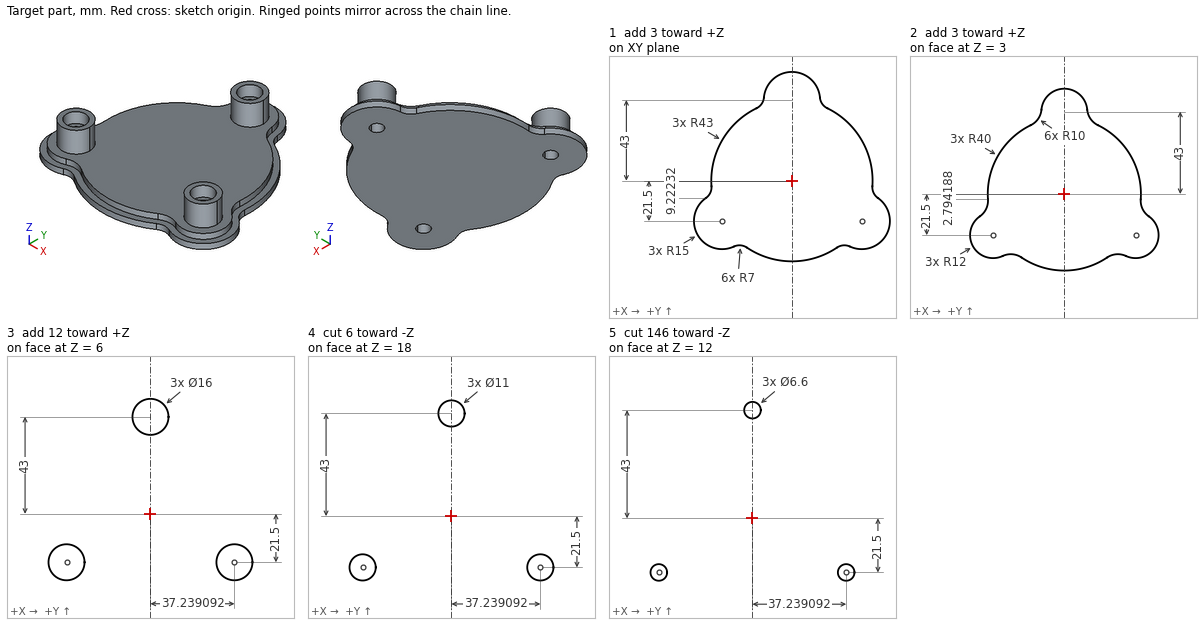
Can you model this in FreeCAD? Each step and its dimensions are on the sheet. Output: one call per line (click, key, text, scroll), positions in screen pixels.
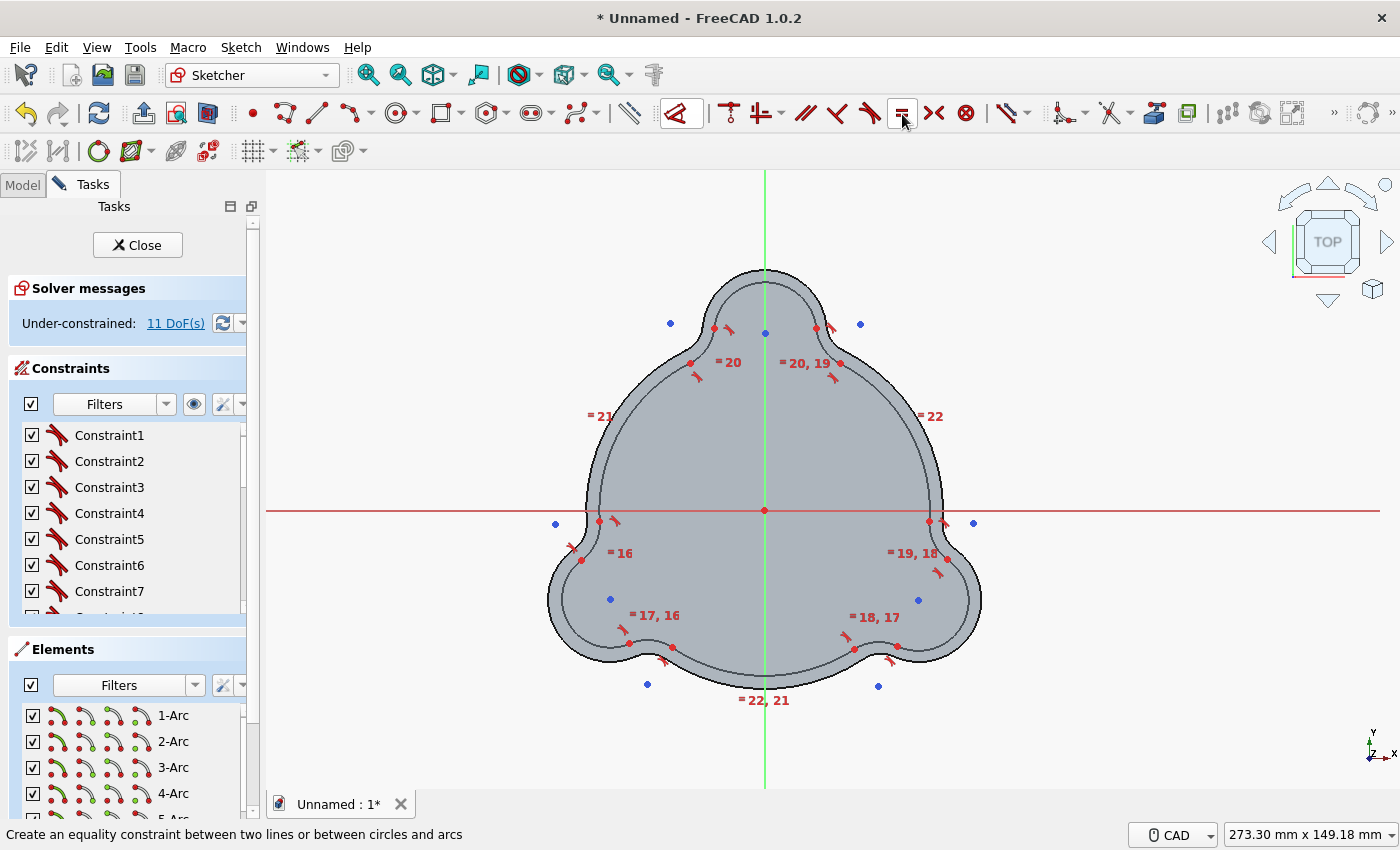
click(562, 596)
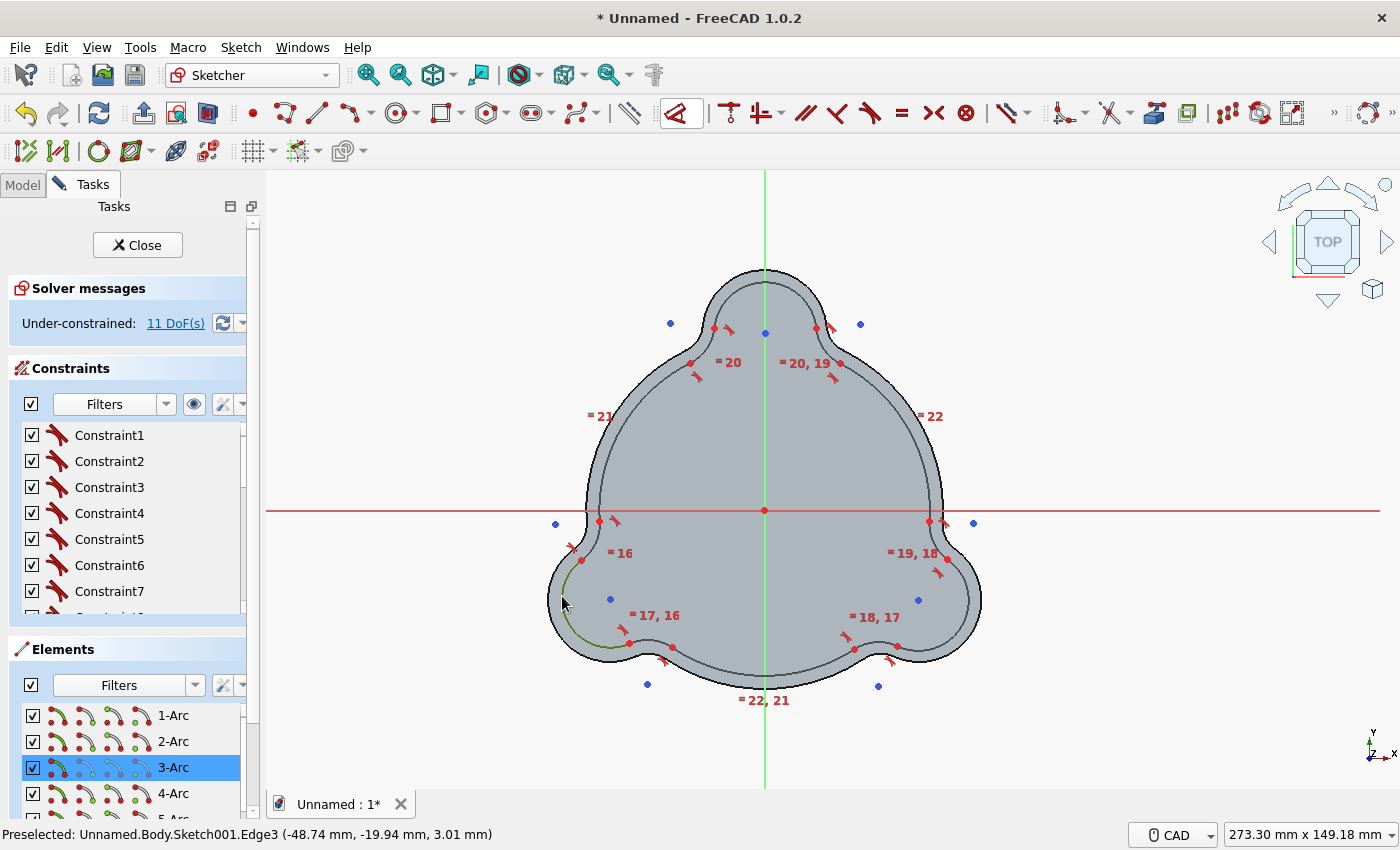
click(940, 646)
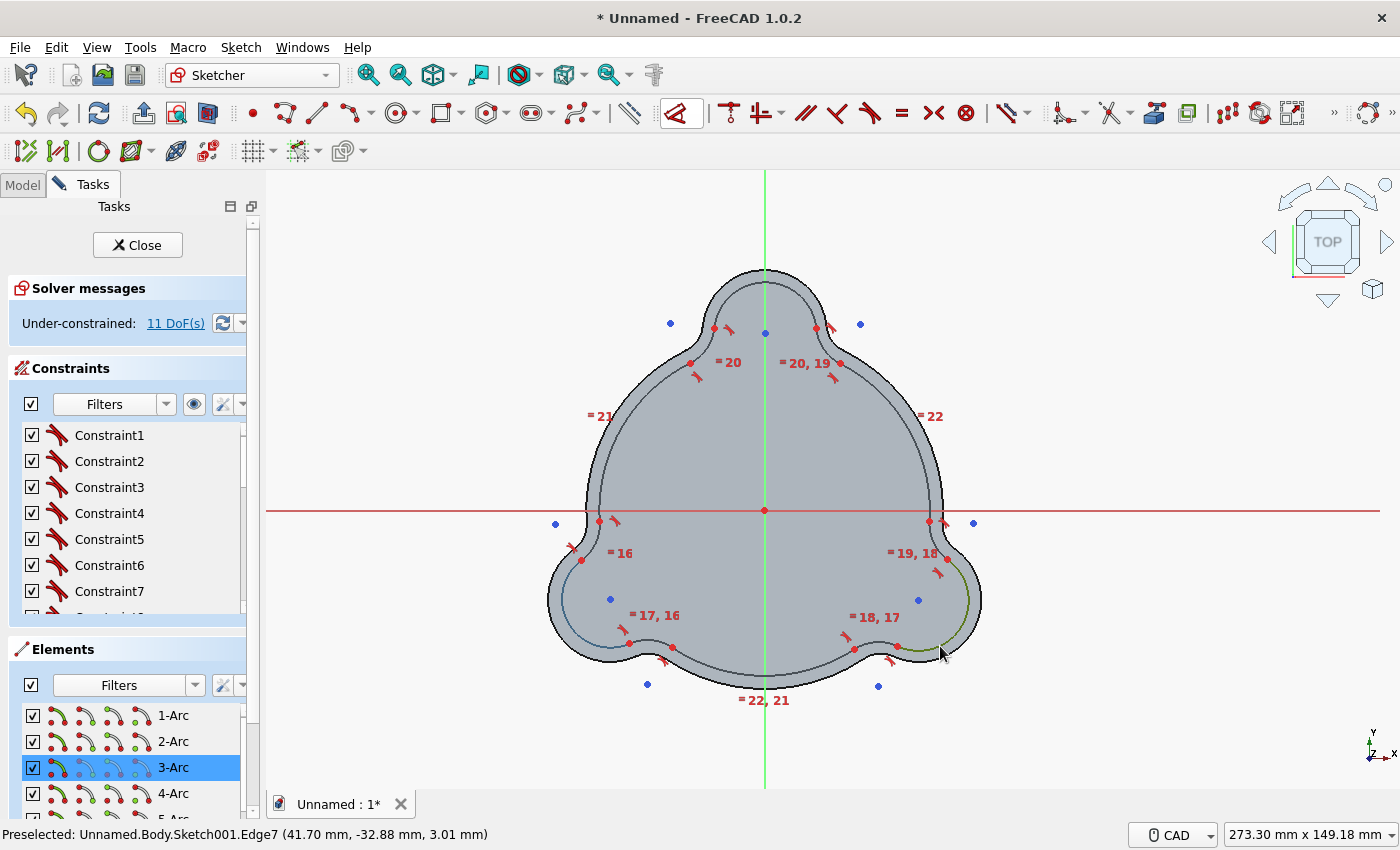
click(794, 291)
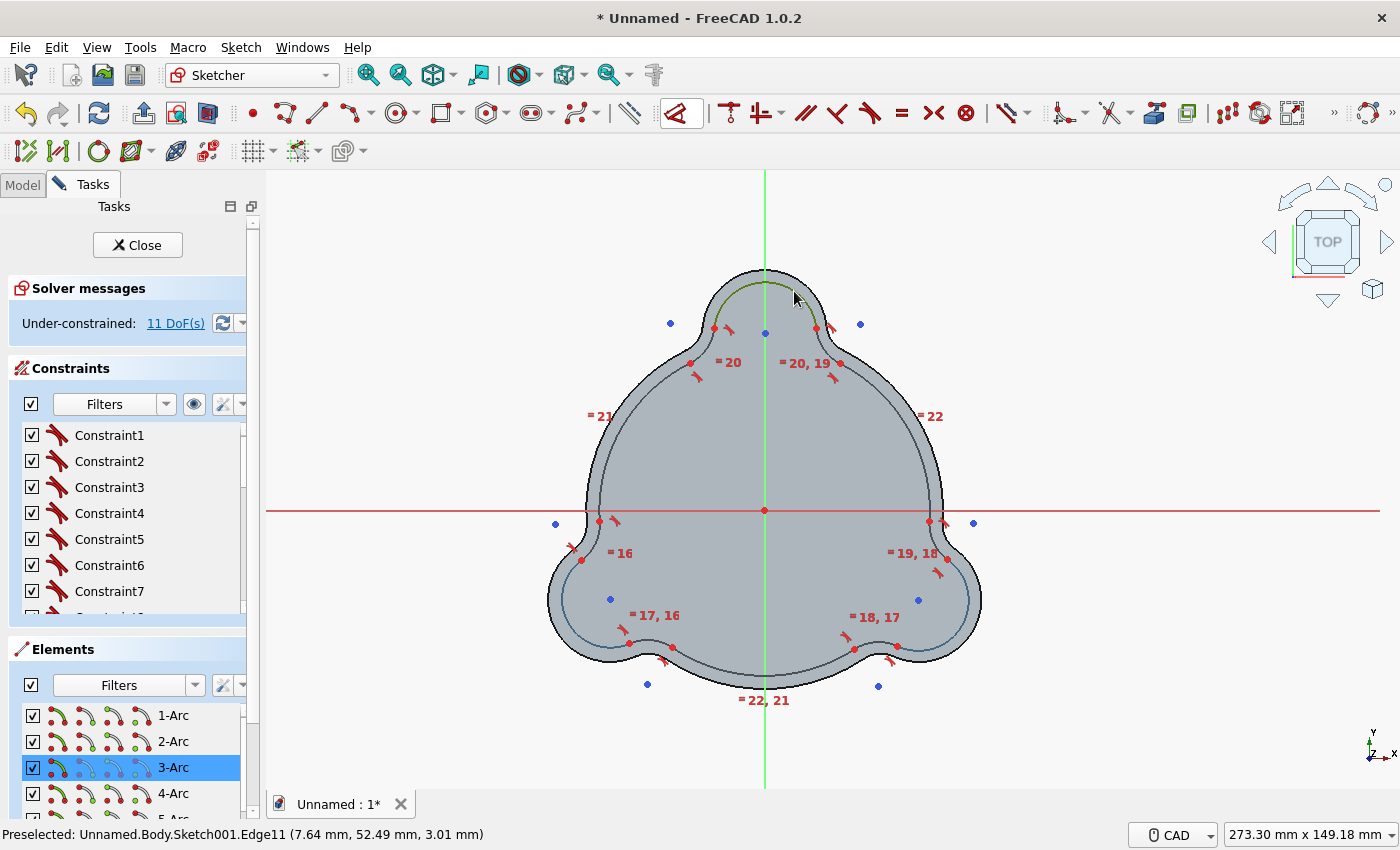
click(902, 114)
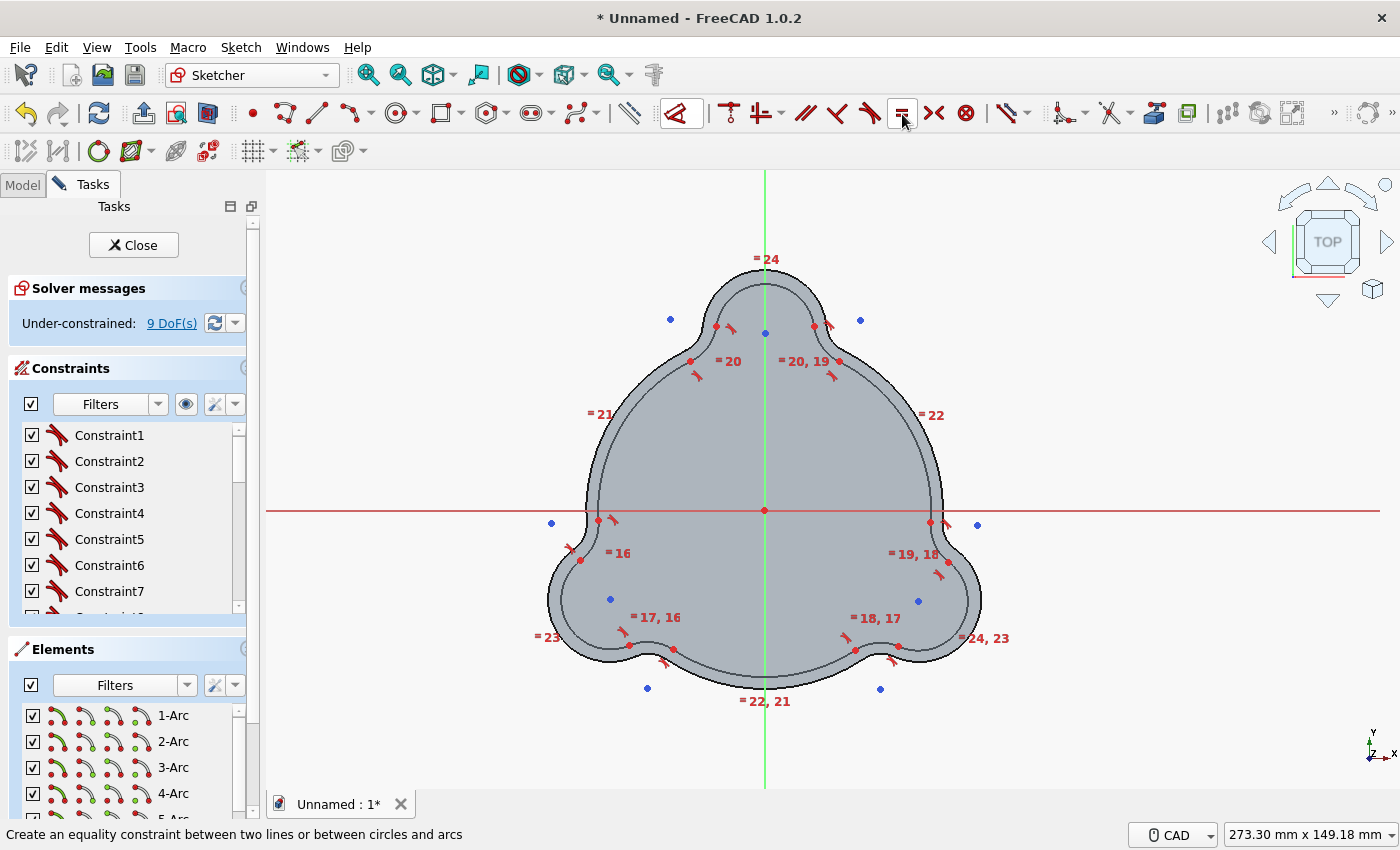
click(765, 334)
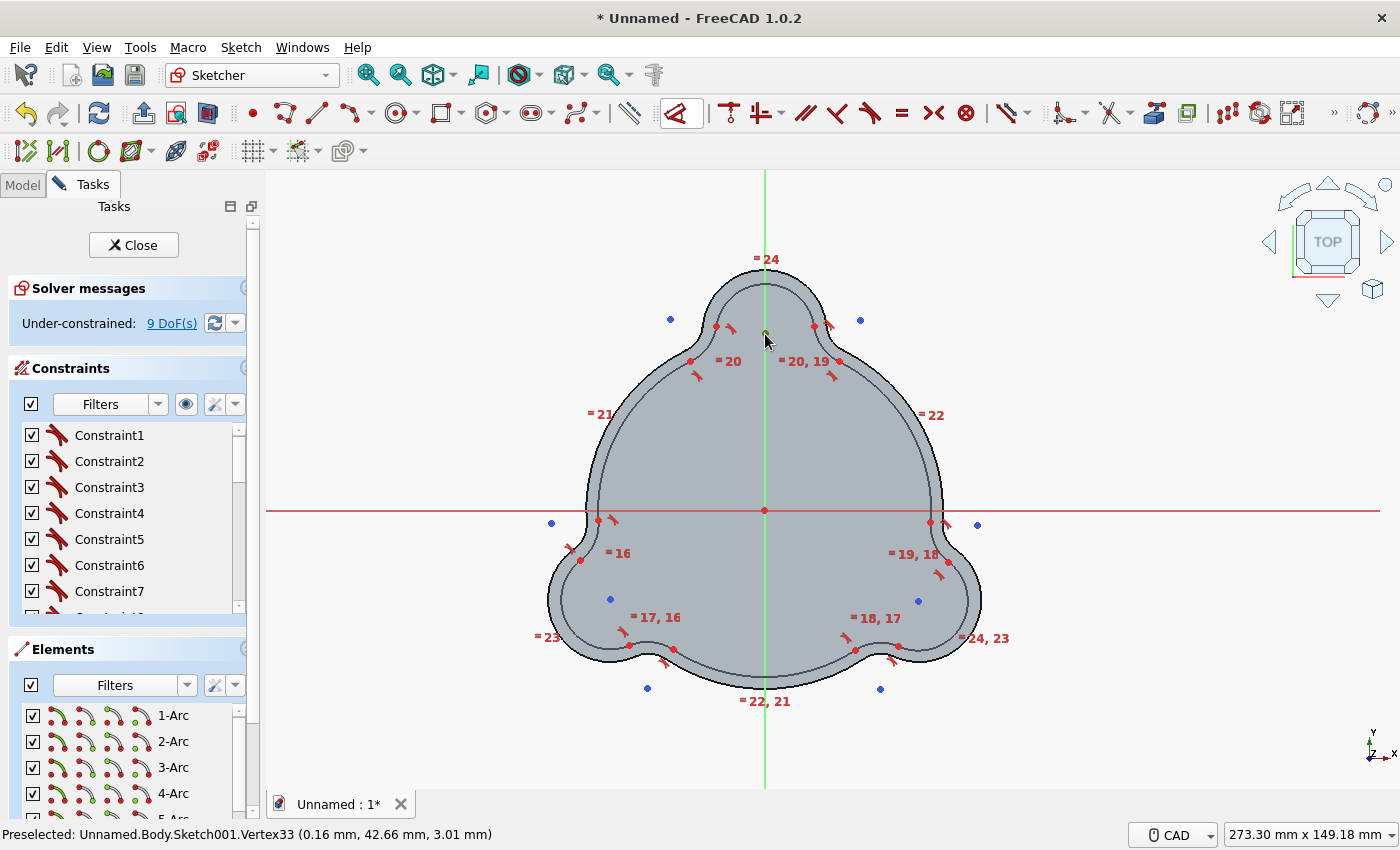
click(765, 721)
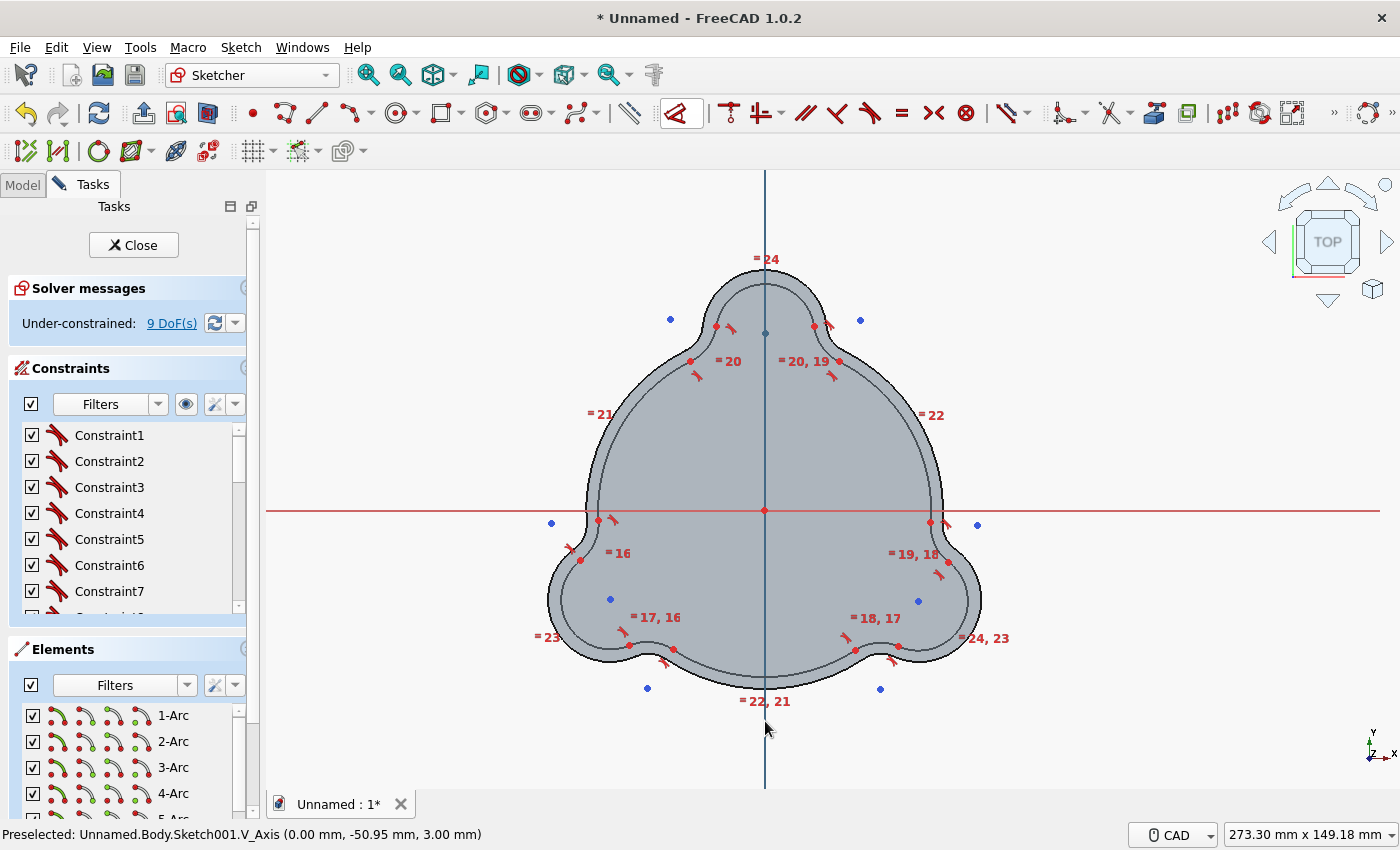
click(730, 114)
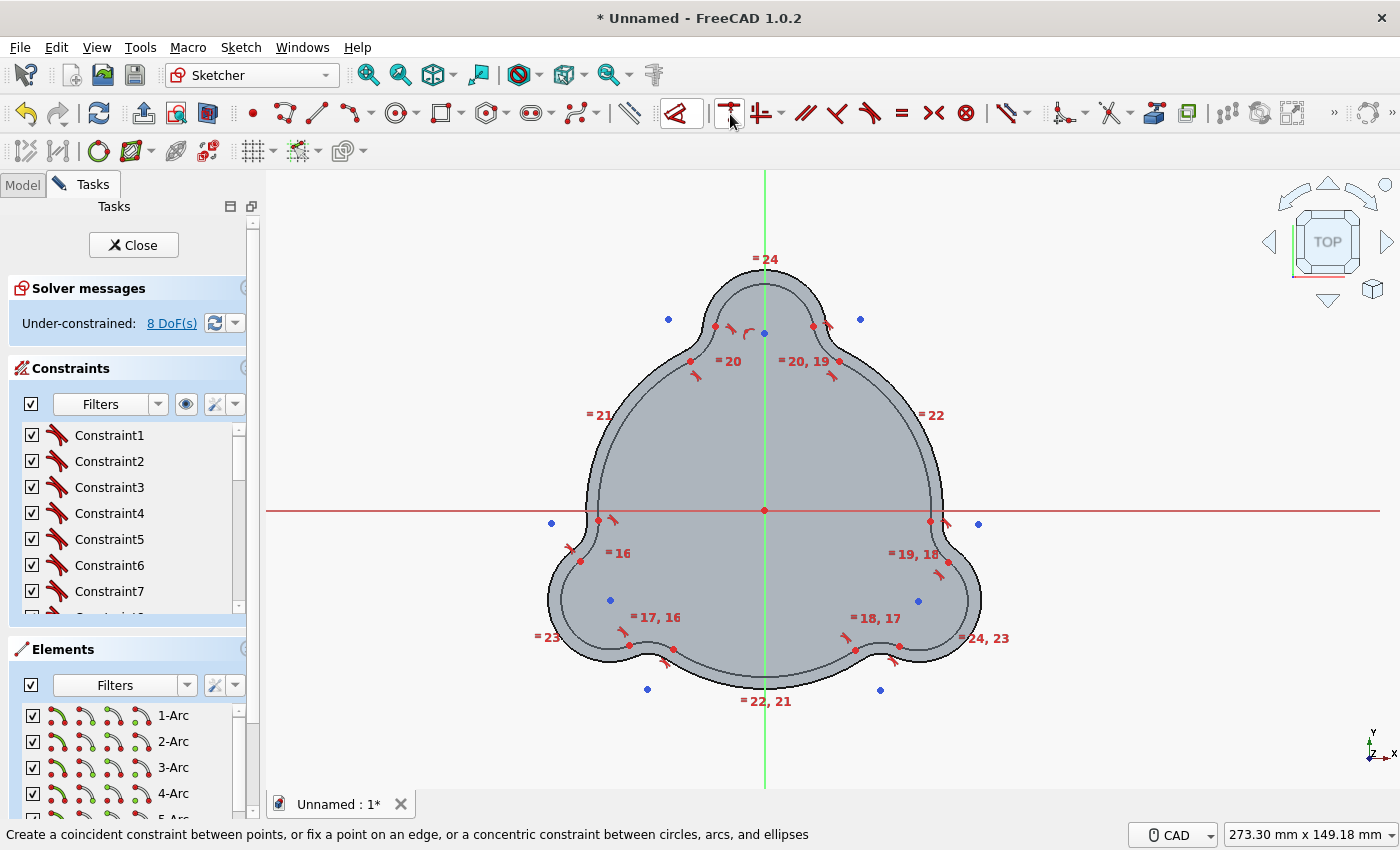
click(611, 600)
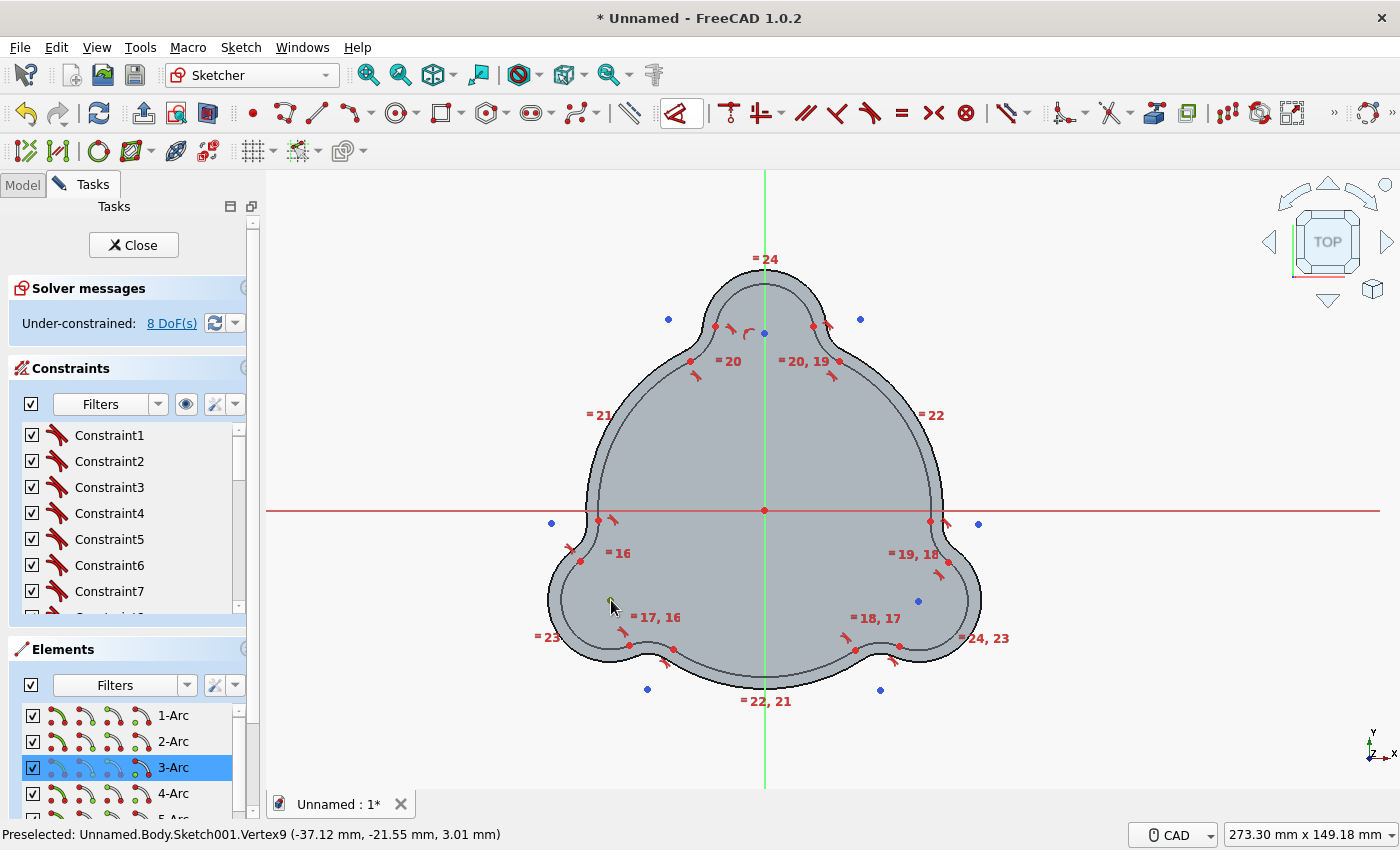
click(918, 601)